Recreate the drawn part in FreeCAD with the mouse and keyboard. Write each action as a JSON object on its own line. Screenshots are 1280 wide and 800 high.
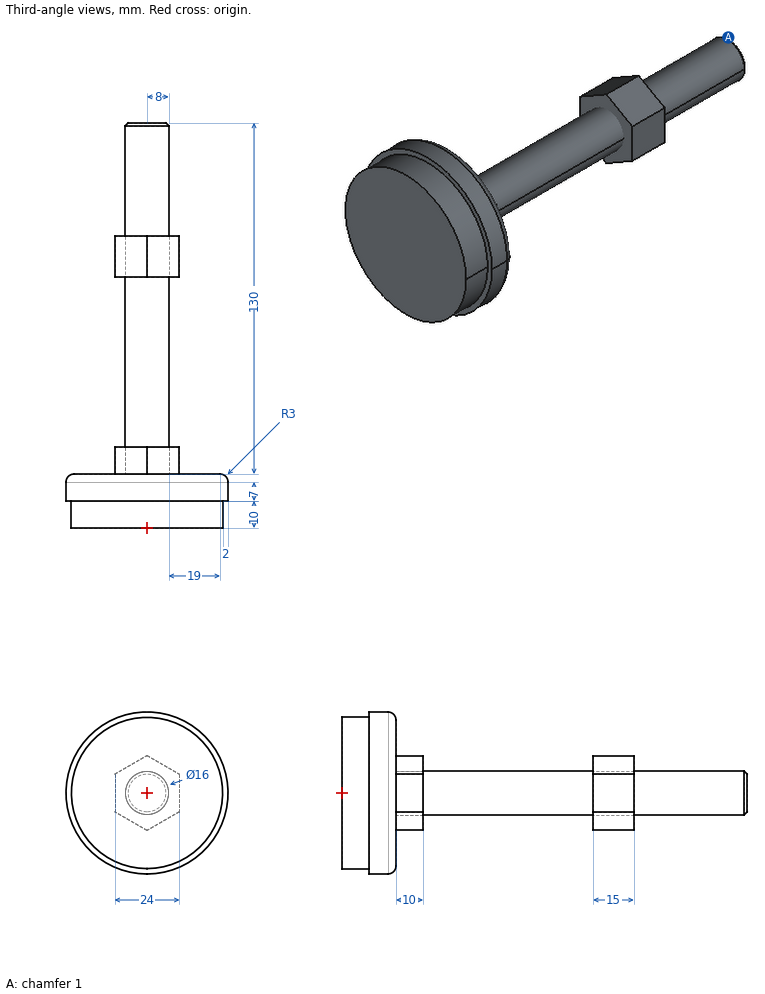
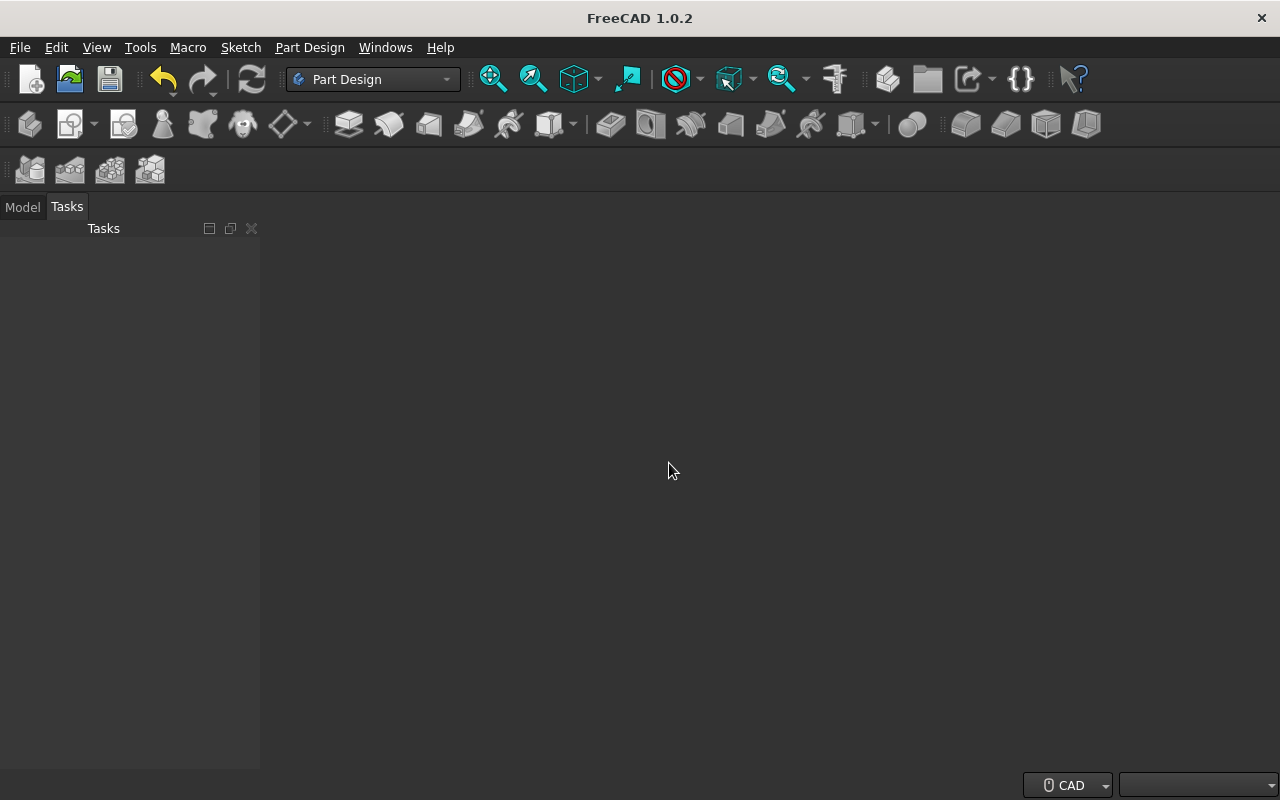
{"action": "left_click", "coordinate": [30, 80]}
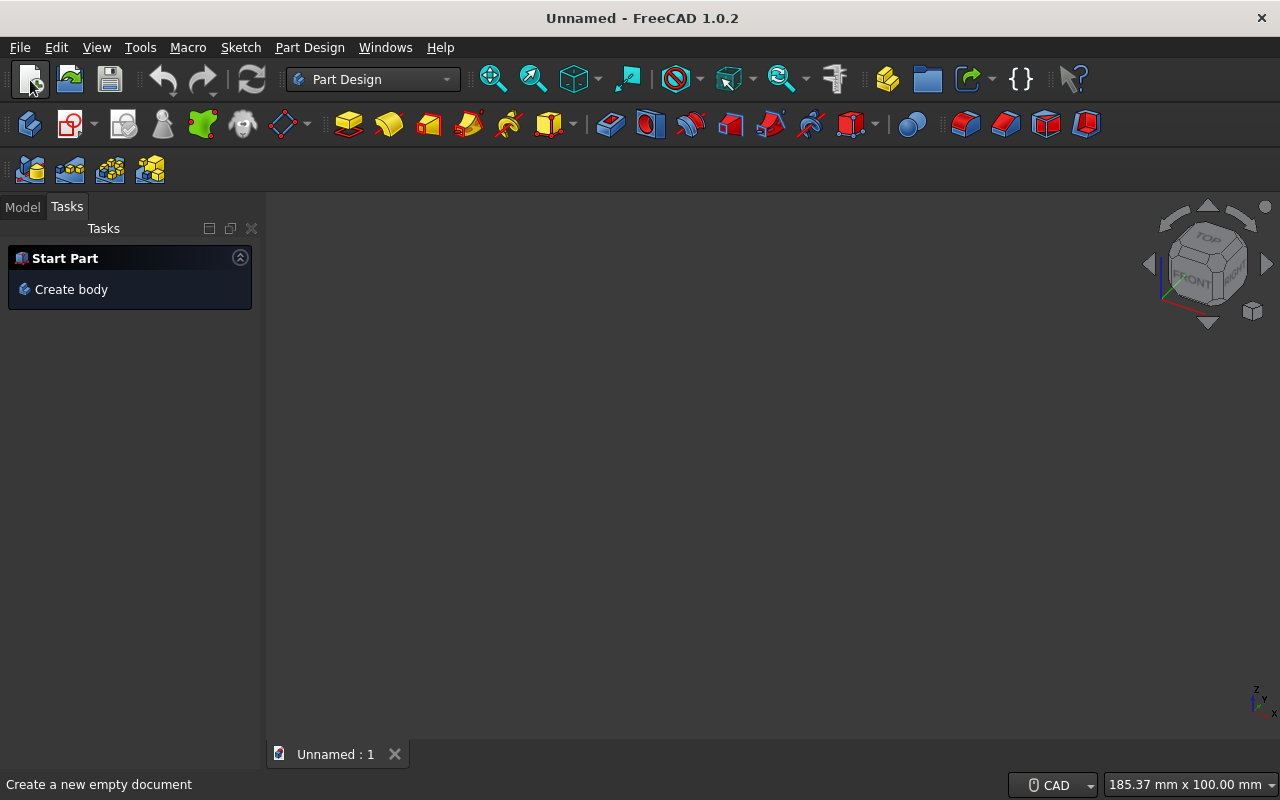
{"action": "left_click", "coordinate": [70, 124]}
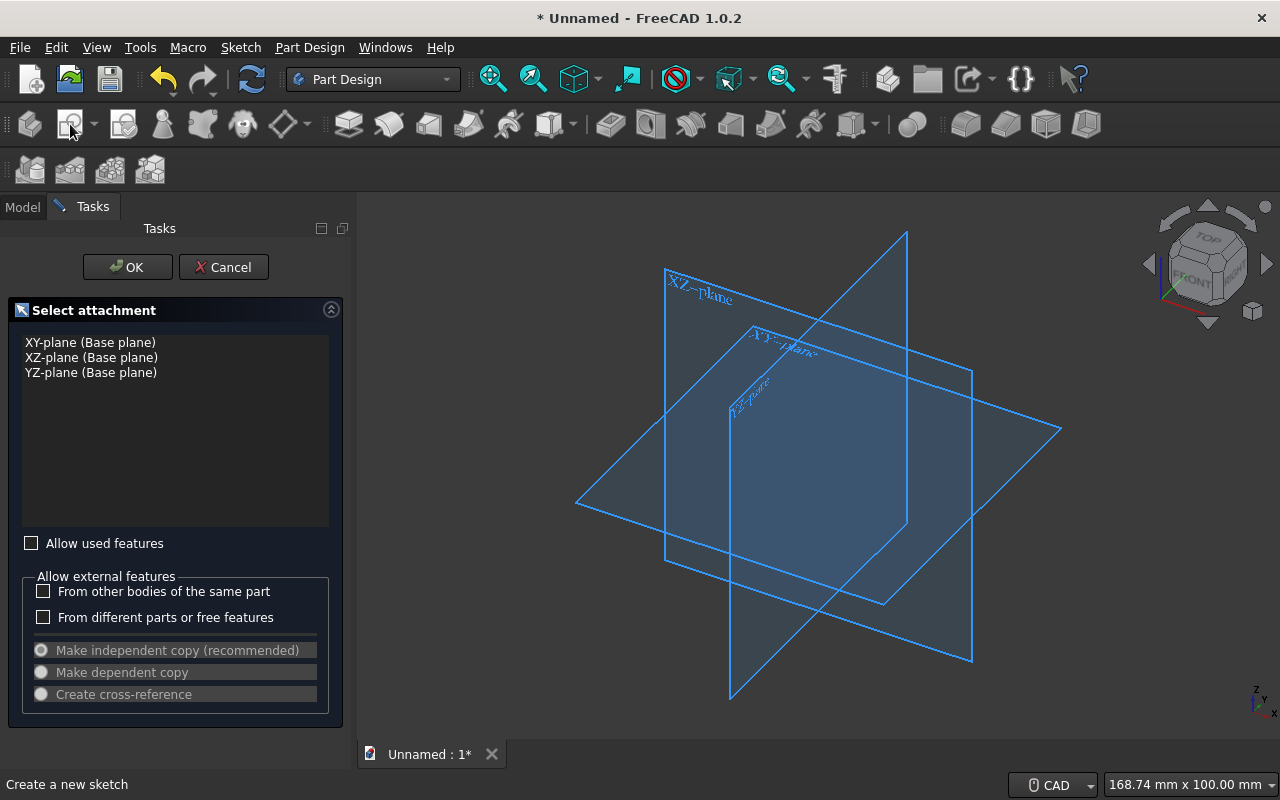
{"action": "left_click", "coordinate": [82, 342]}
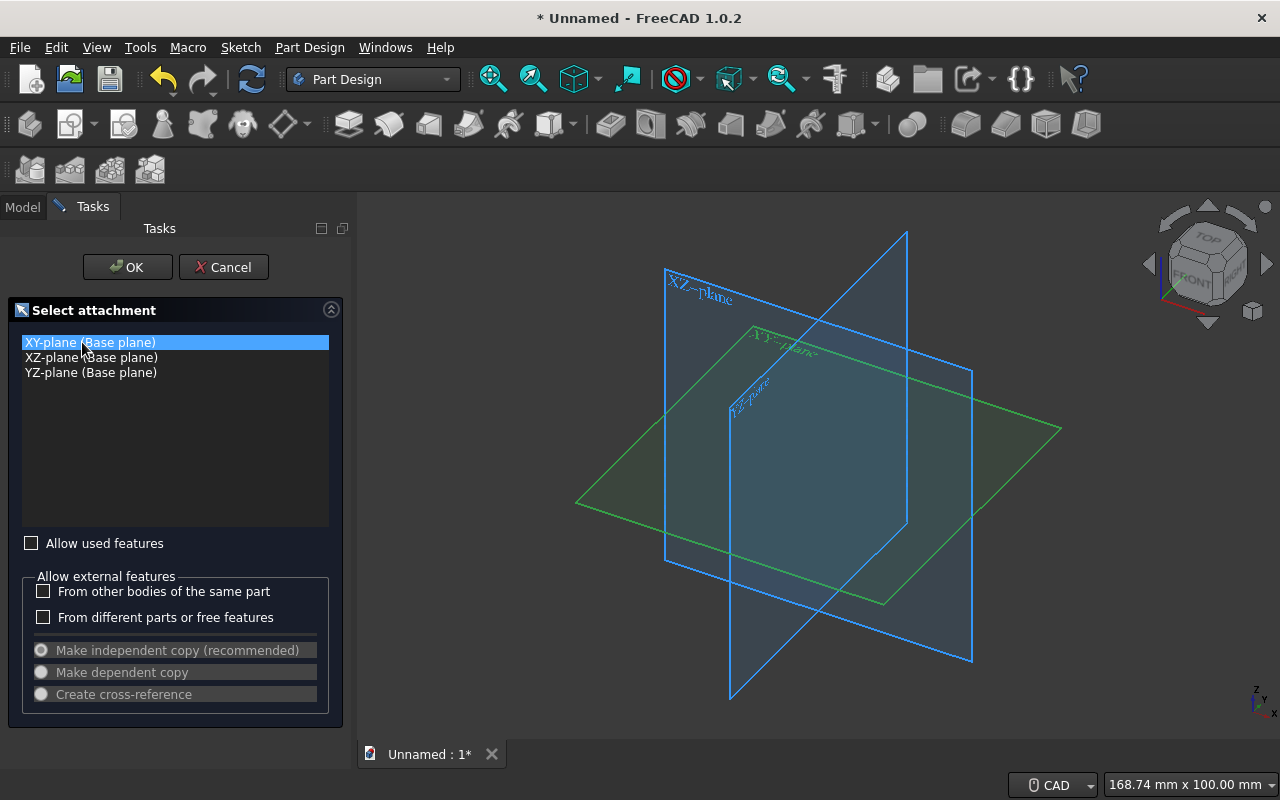
{"action": "left_click", "coordinate": [128, 267]}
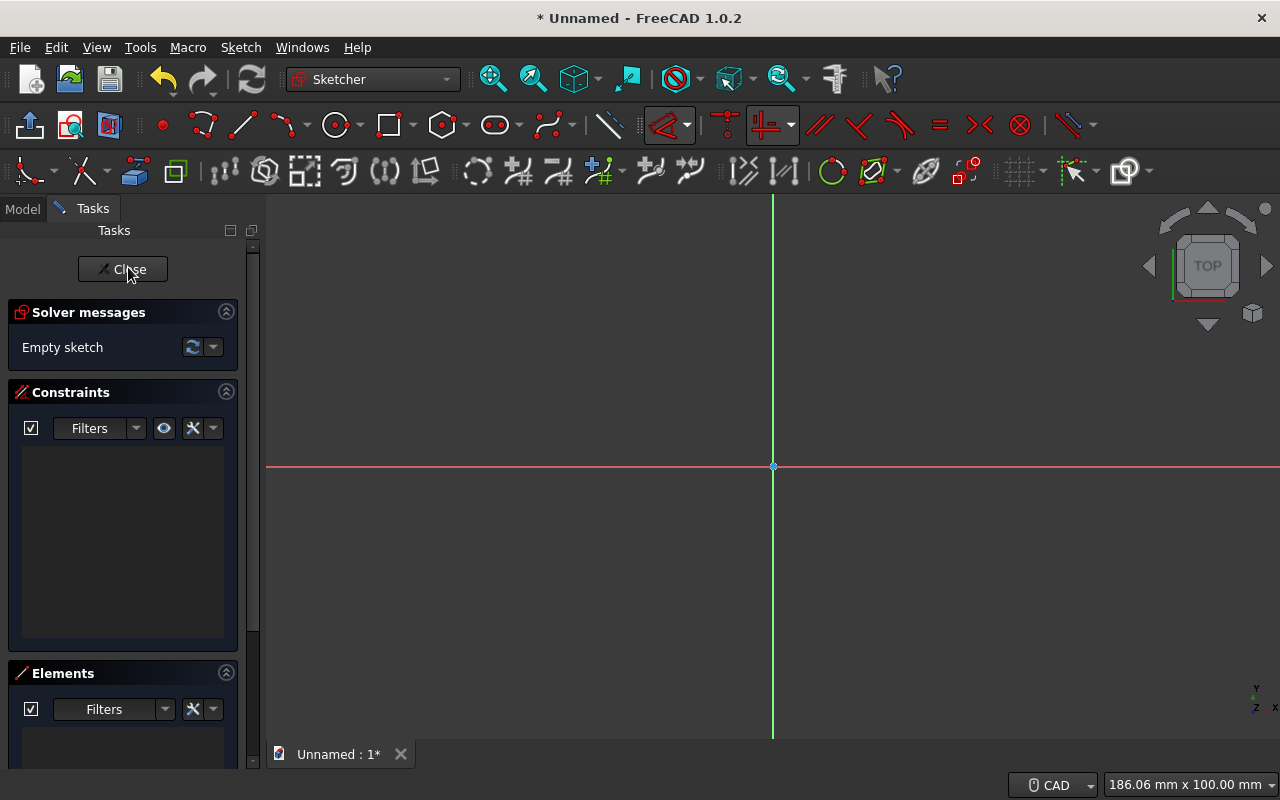
{"action": "scroll", "coordinate": [617, 704], "scroll_direction": "down", "scroll_amount": 5}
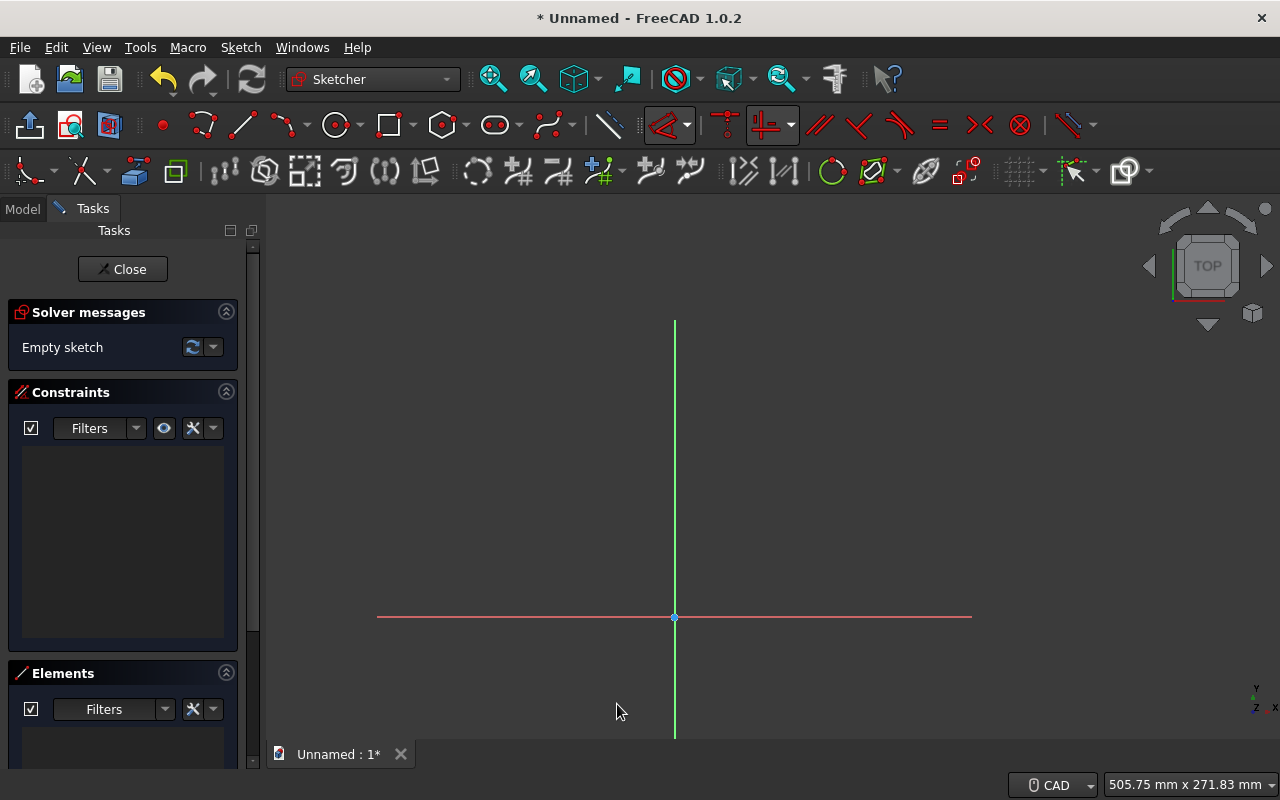
{"action": "left_click", "coordinate": [204, 126]}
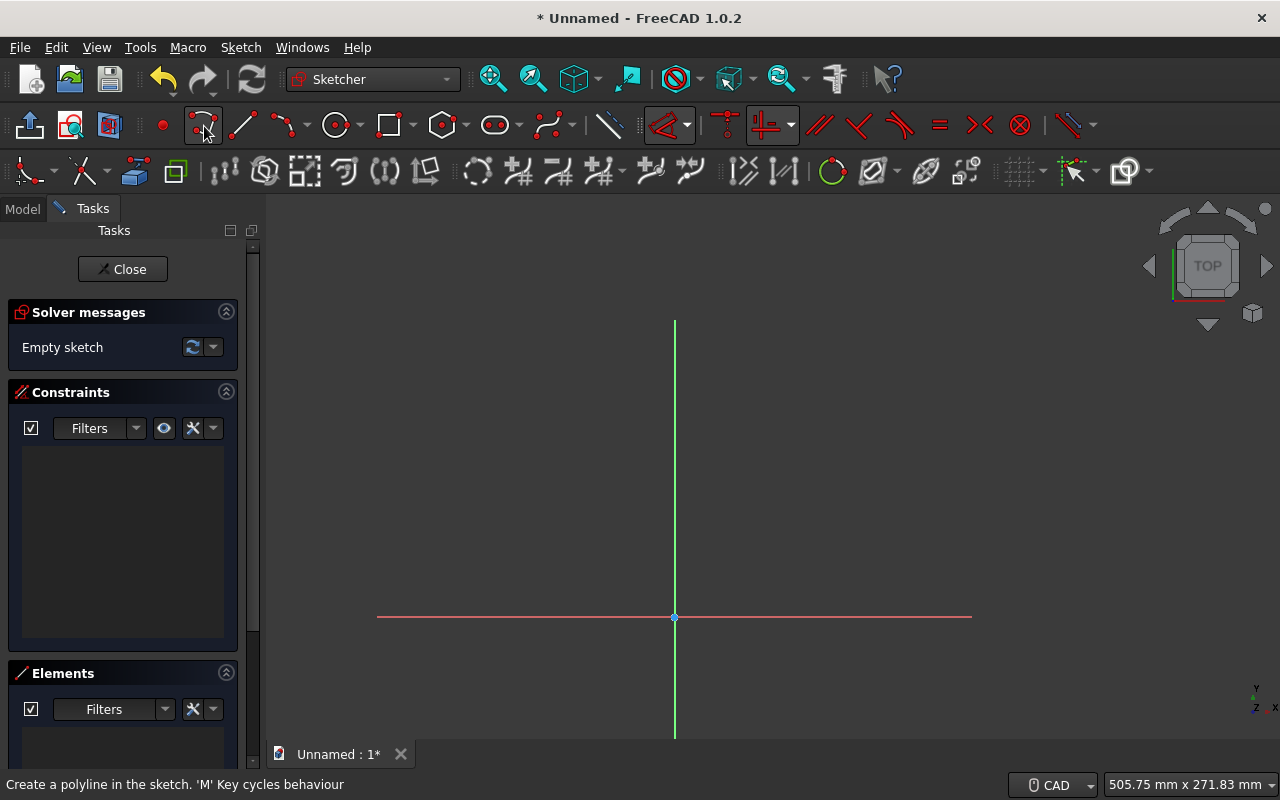
{"action": "left_click", "coordinate": [729, 577]}
{"action": "left_click", "coordinate": [691, 577]}
{"action": "left_click", "coordinate": [691, 316]}
{"action": "left_click", "coordinate": [675, 316]}
{"action": "left_click", "coordinate": [675, 617]}
{"action": "left_click", "coordinate": [731, 608]}
{"action": "left_click", "coordinate": [731, 597]}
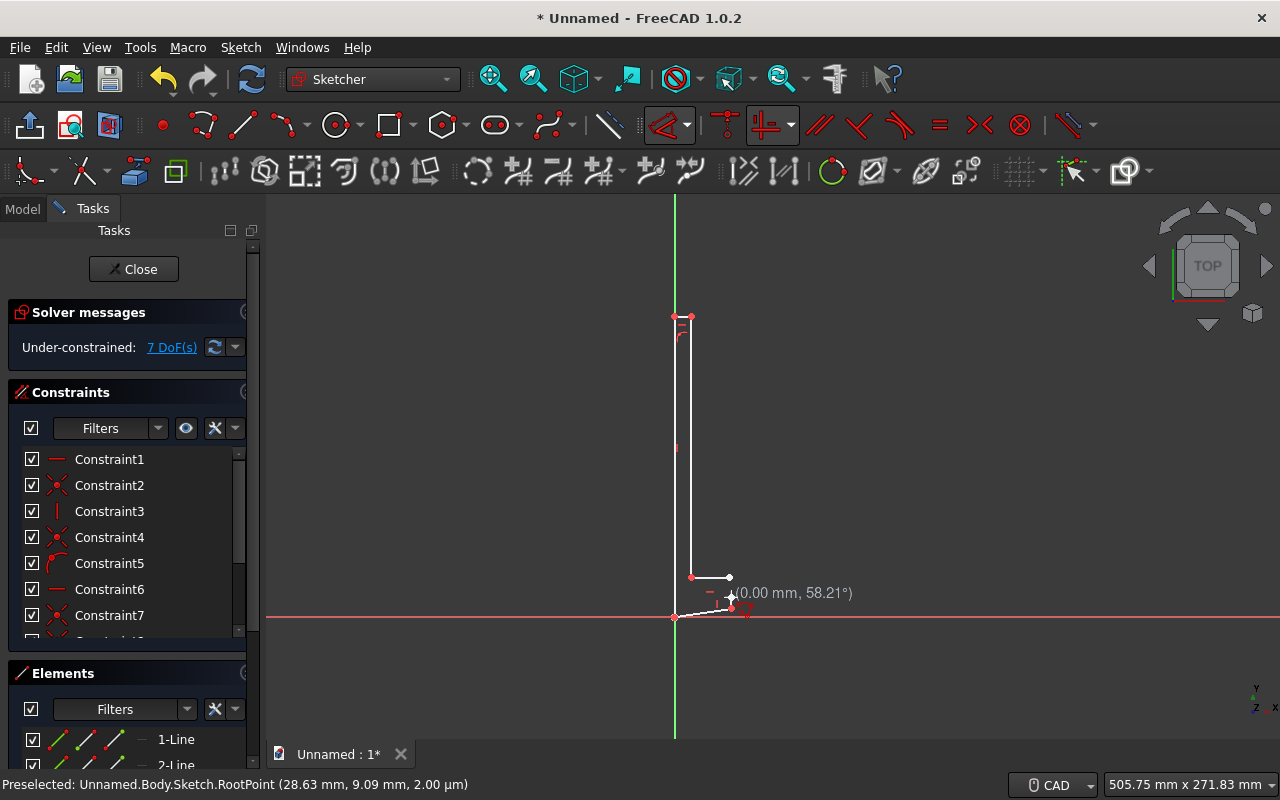
{"action": "scroll", "coordinate": [735, 597], "scroll_direction": "up", "scroll_amount": 7}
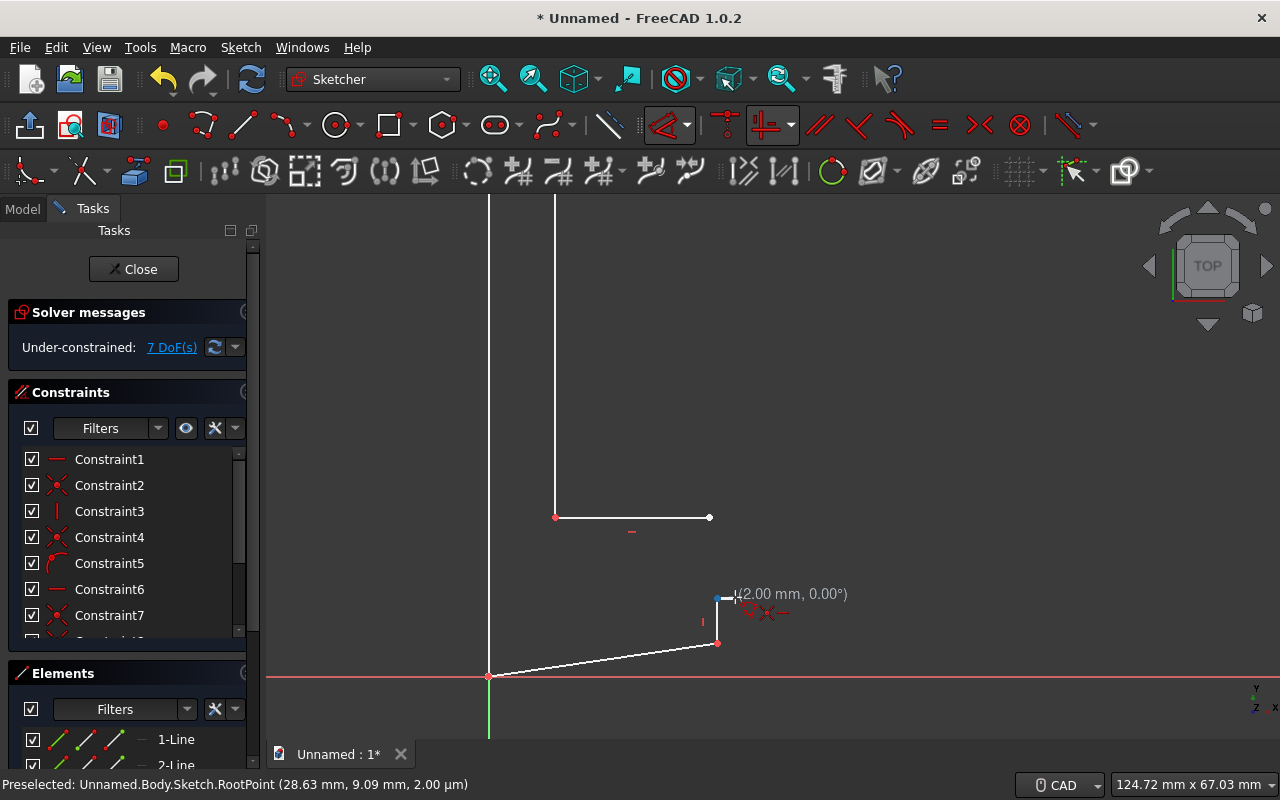
{"action": "left_click", "coordinate": [733, 595]}
{"action": "left_click", "coordinate": [733, 539]}
{"action": "right_click", "coordinate": [733, 539]}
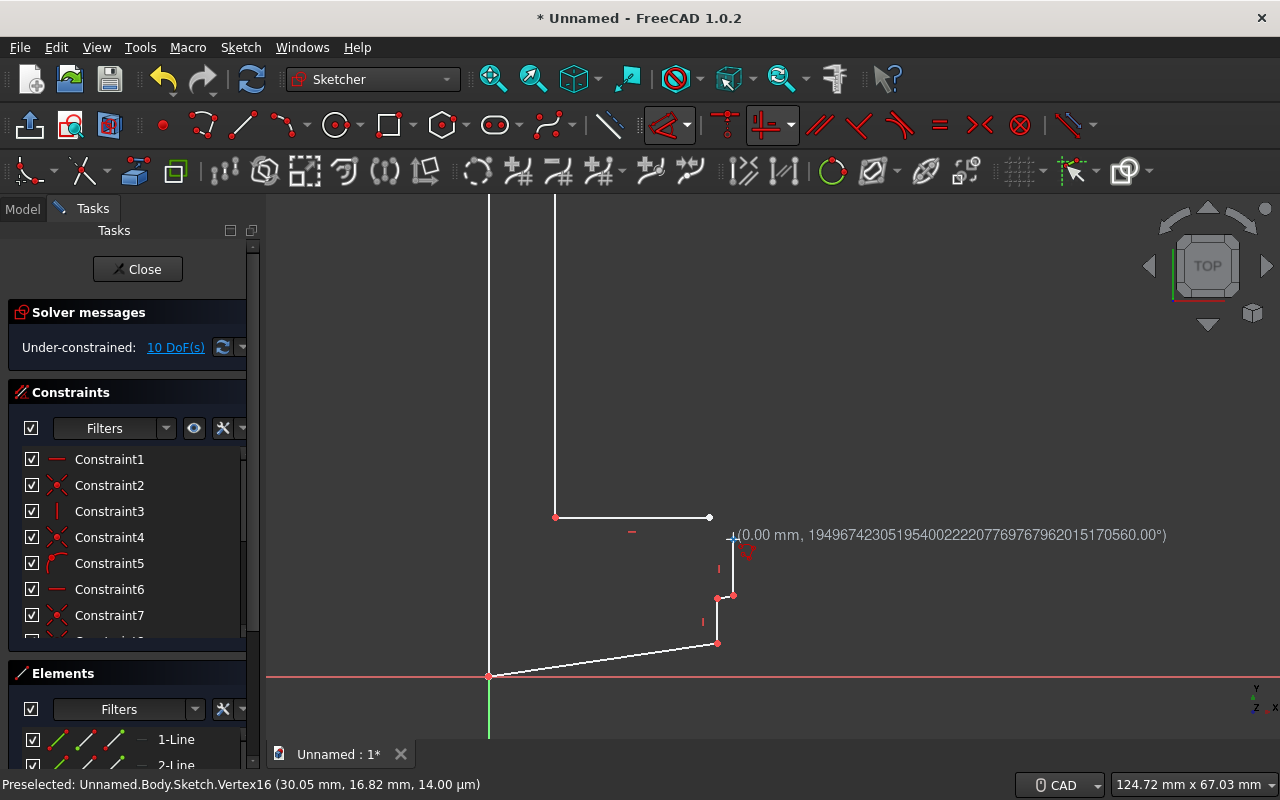
{"action": "left_click", "coordinate": [284, 126]}